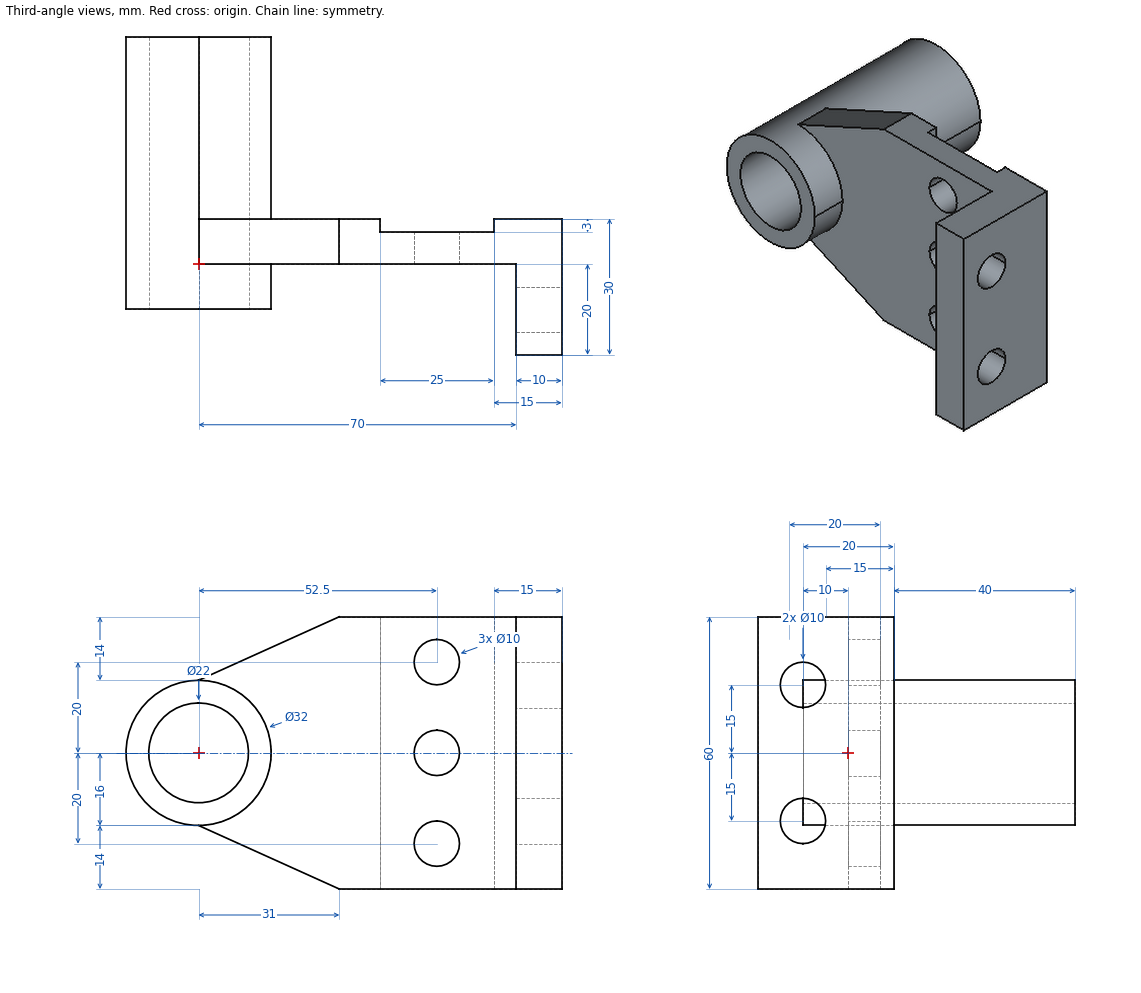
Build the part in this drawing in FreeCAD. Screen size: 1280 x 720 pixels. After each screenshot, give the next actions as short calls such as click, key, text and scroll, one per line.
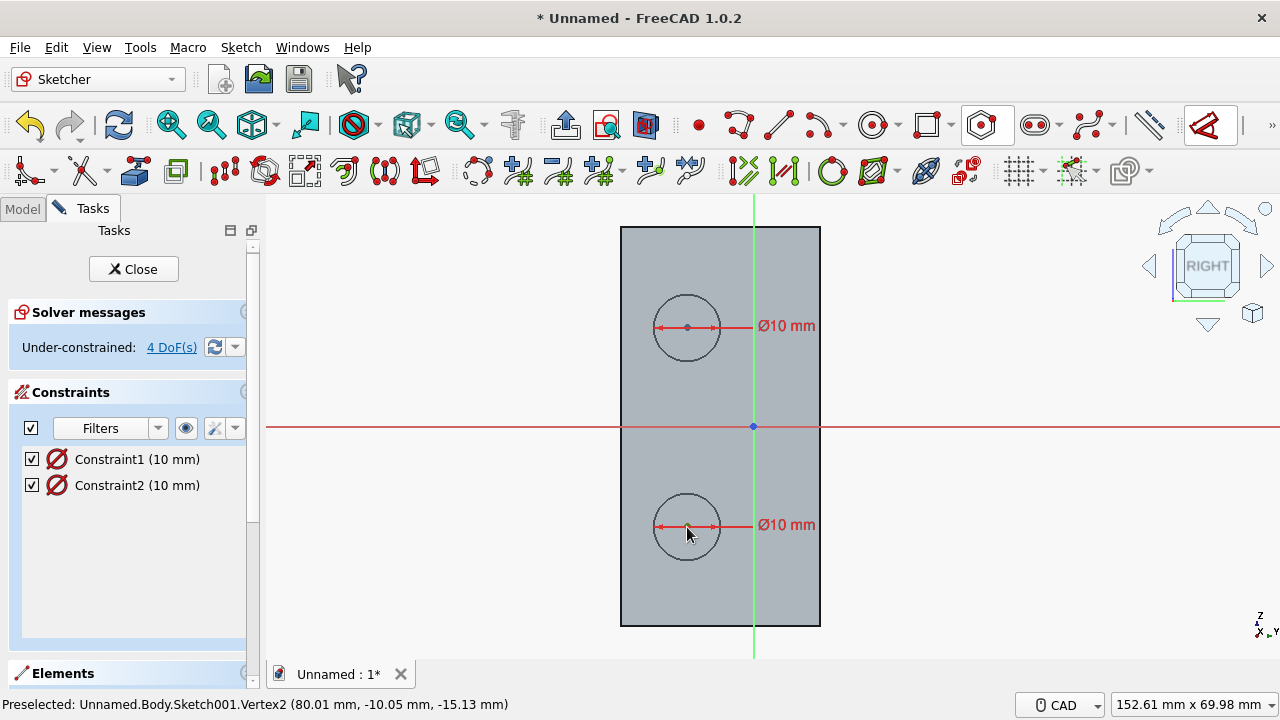
key(v)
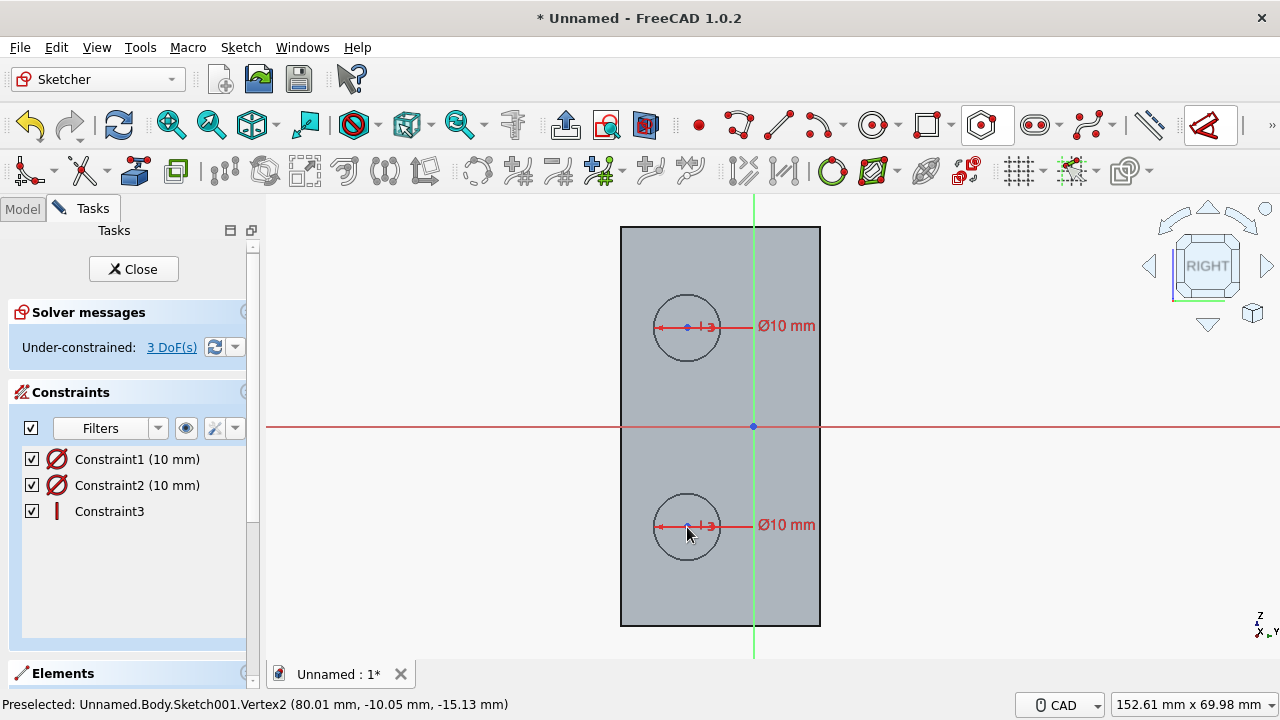
click(687, 328)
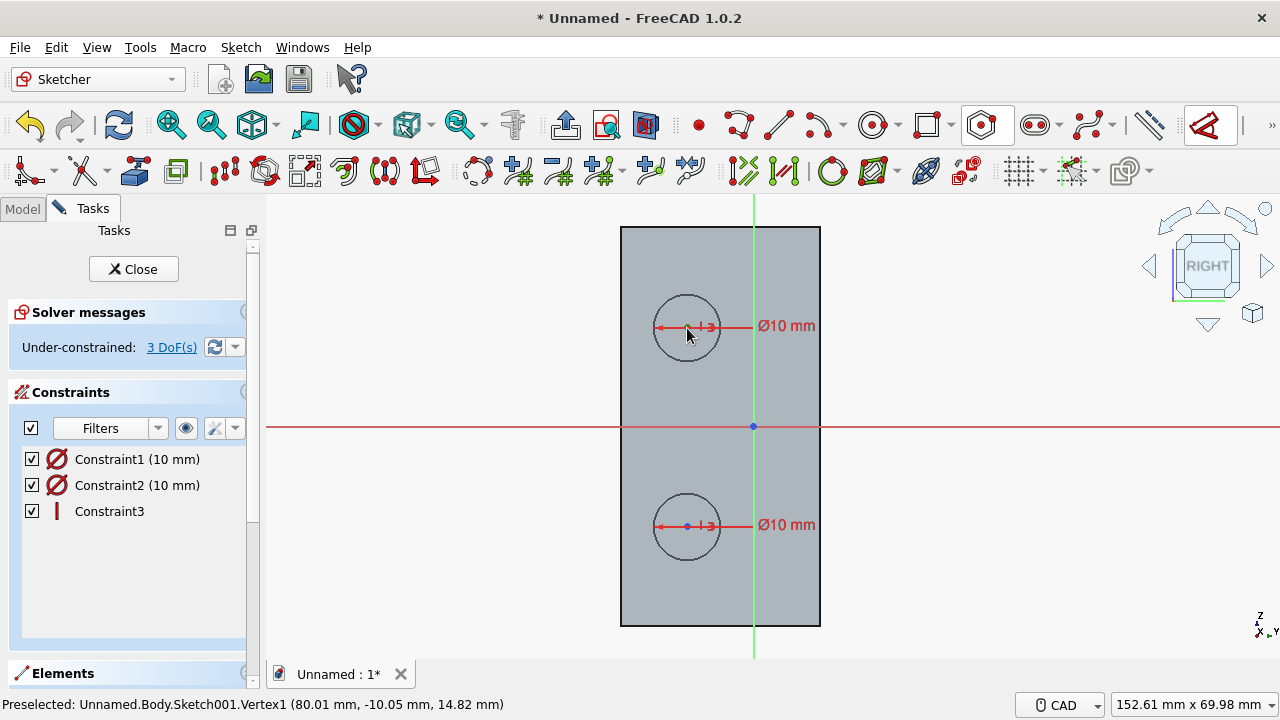
key(l)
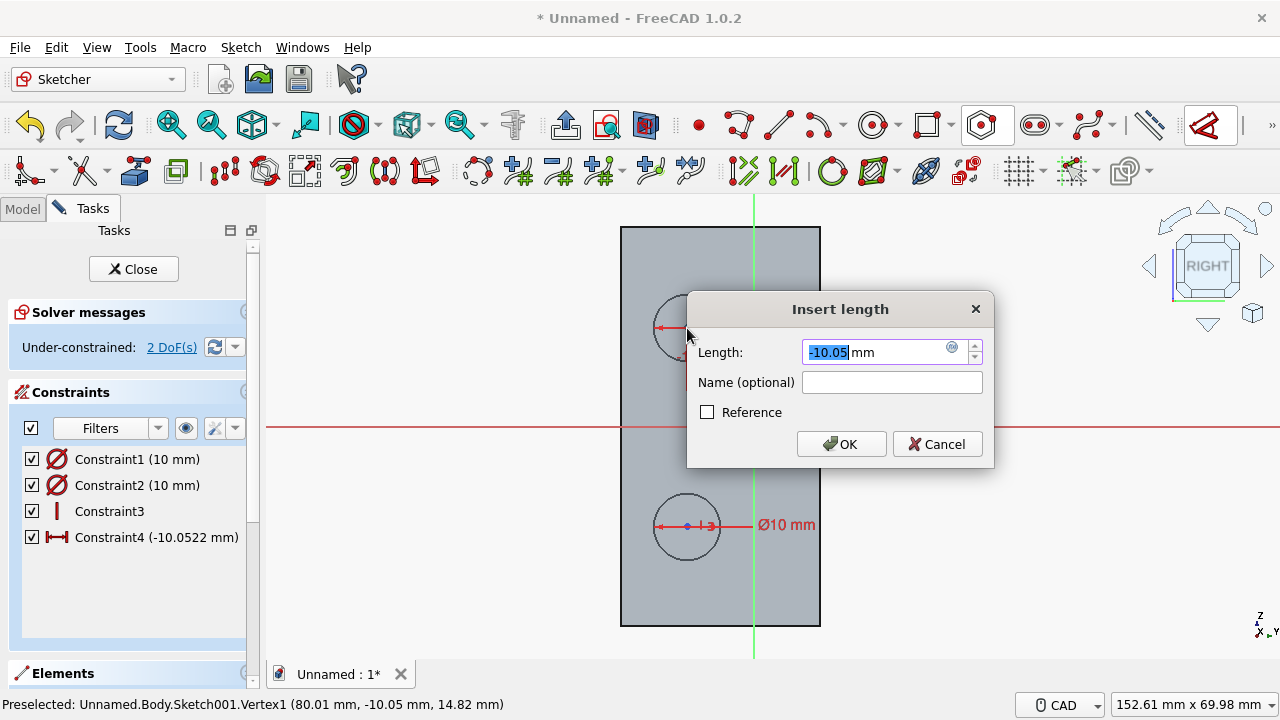
text(-10)
key(Return)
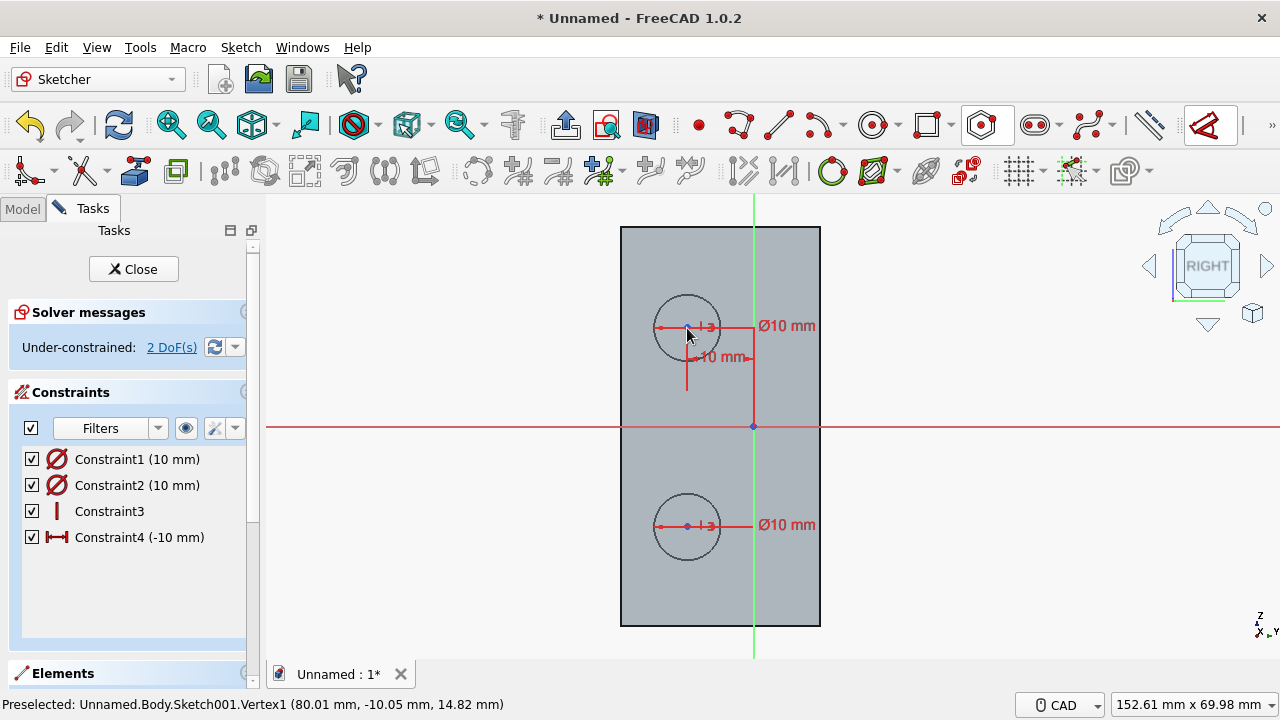
click(687, 328)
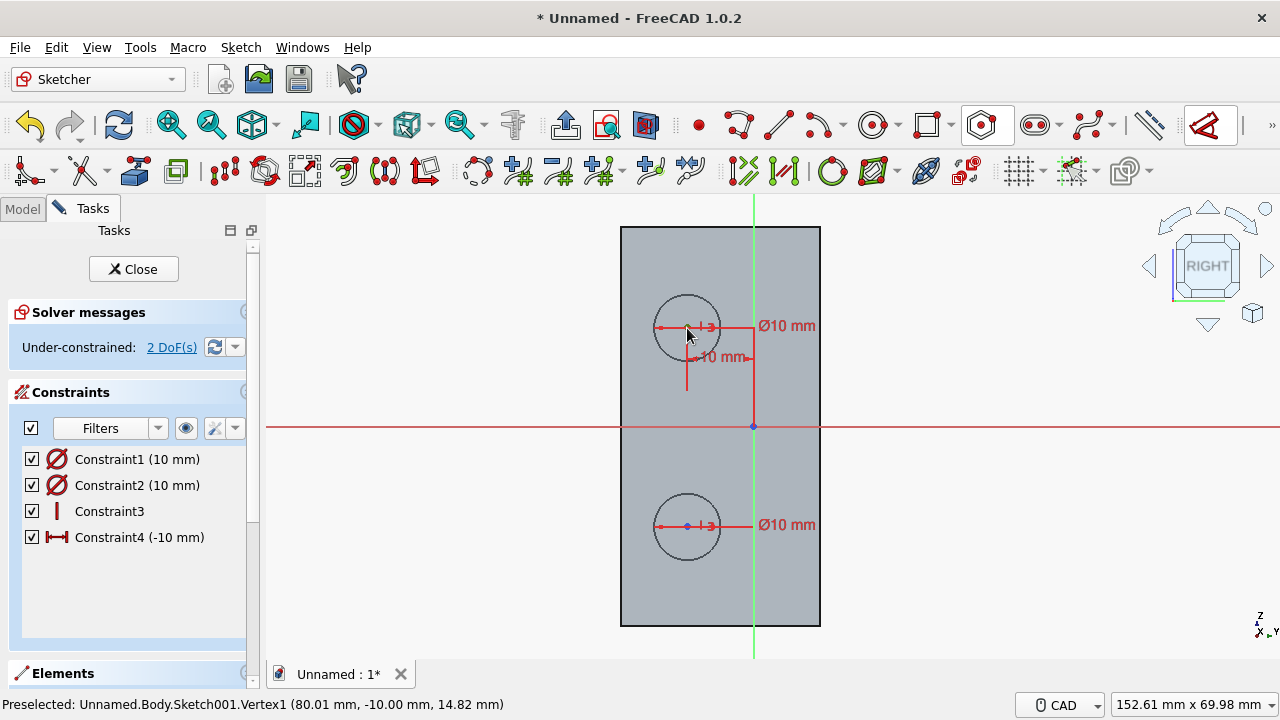
click(1232, 126)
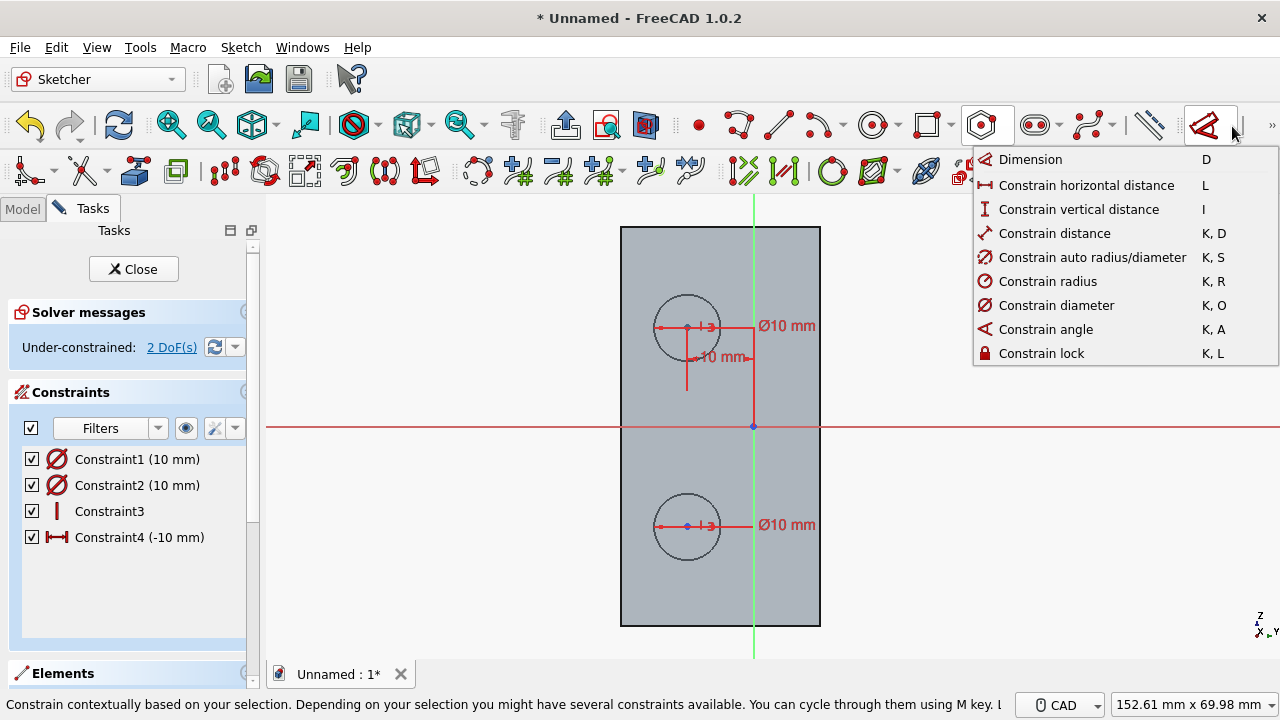
click(1126, 209)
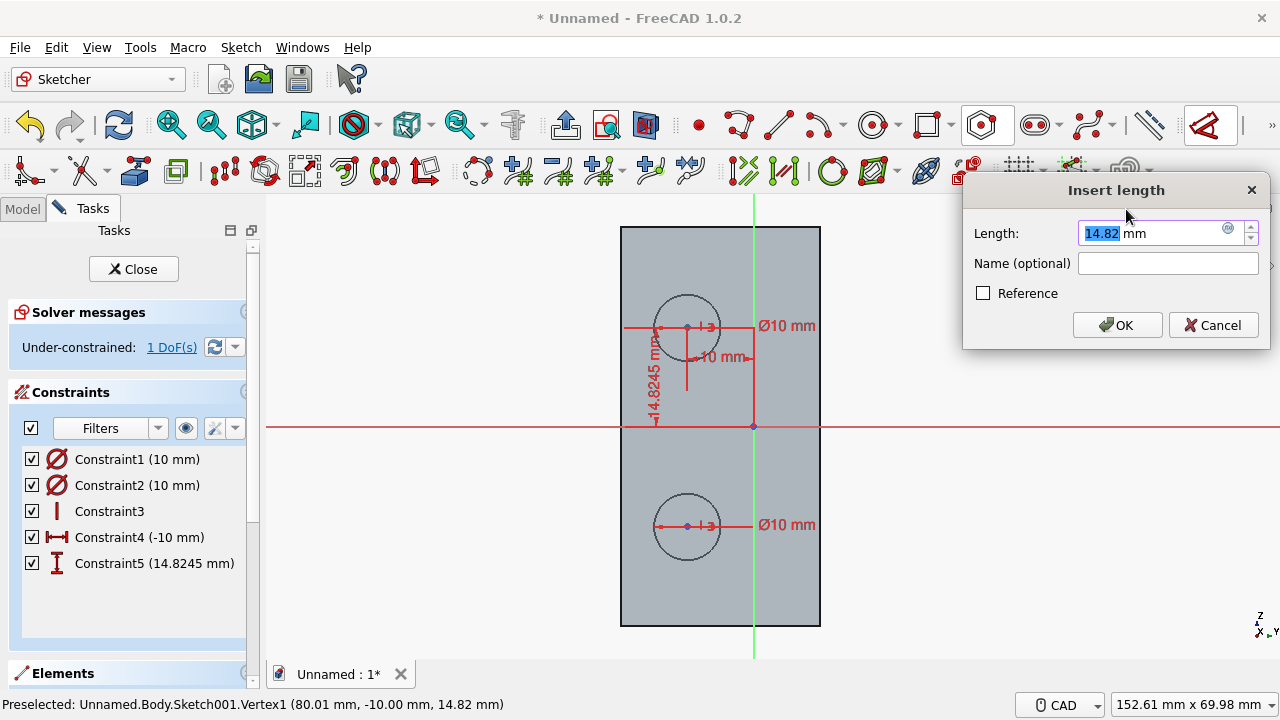
text(15)
key(Return)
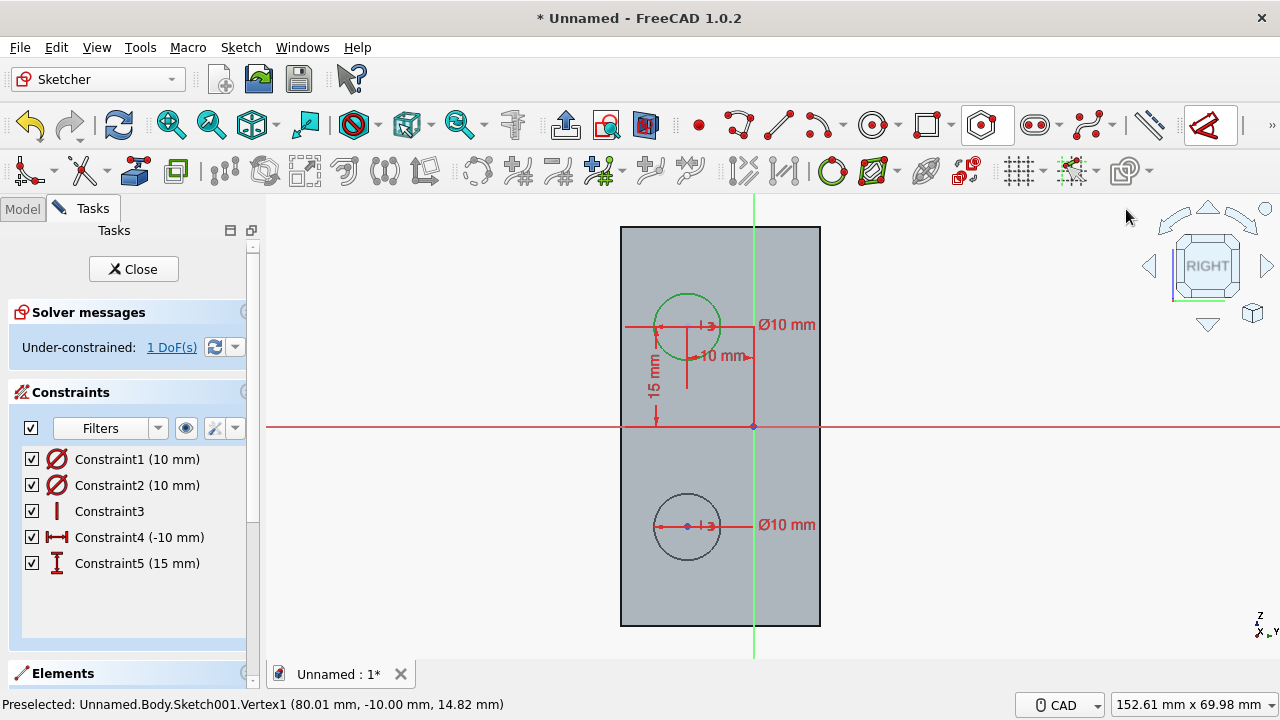
click(687, 527)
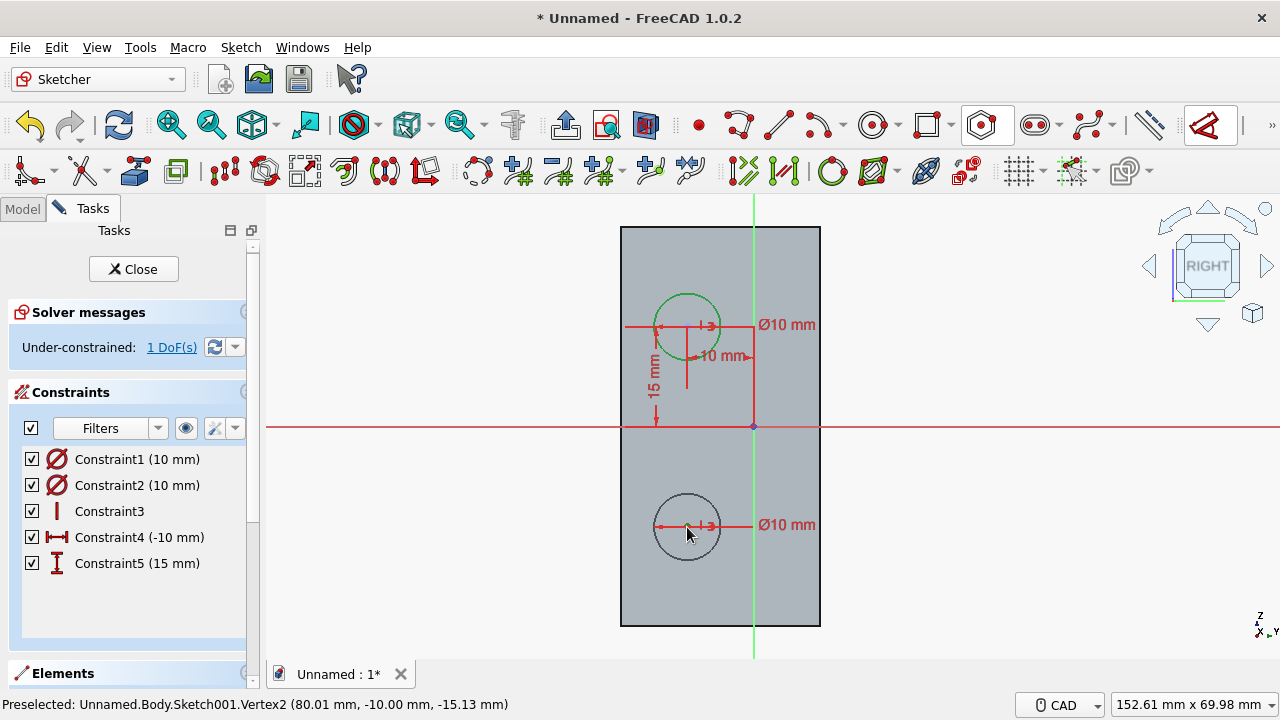
click(1232, 126)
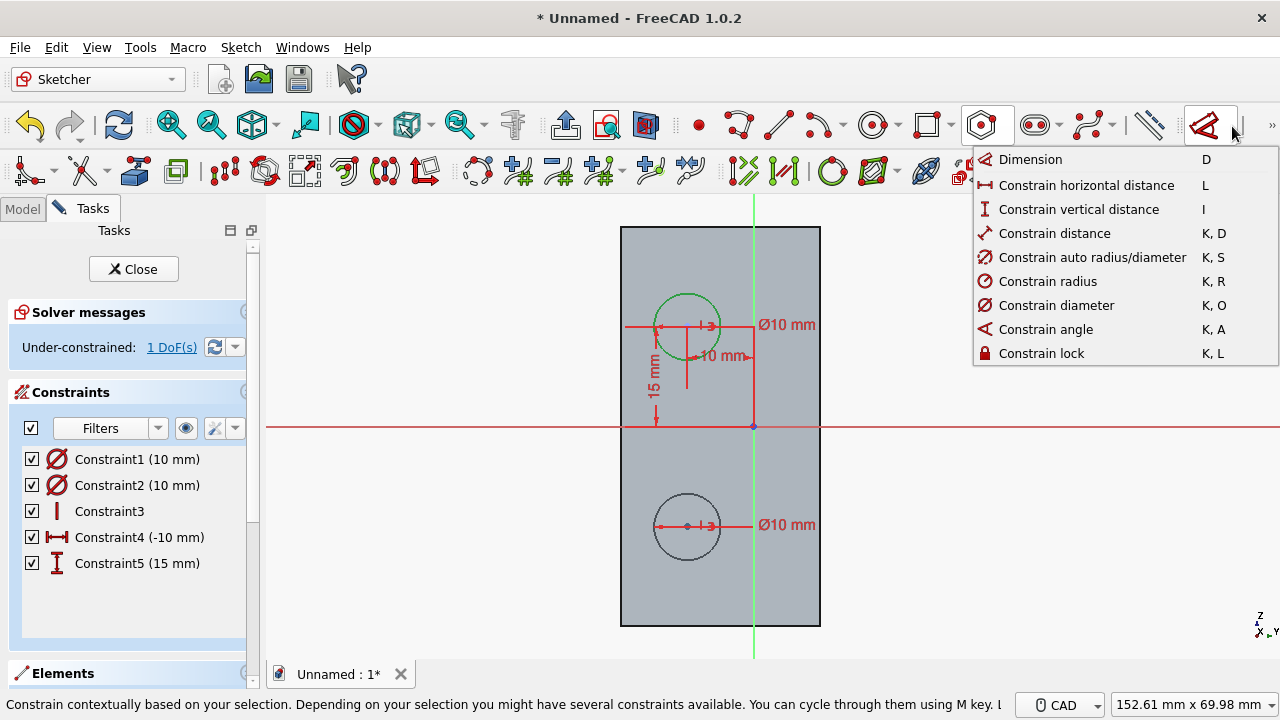
click(1126, 209)